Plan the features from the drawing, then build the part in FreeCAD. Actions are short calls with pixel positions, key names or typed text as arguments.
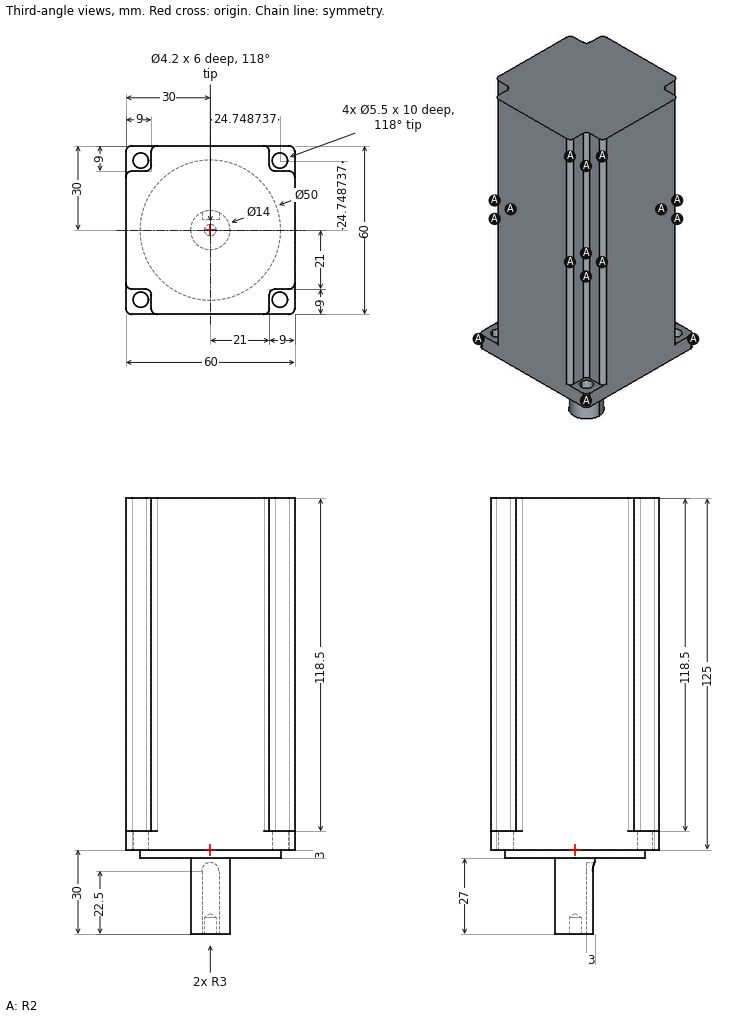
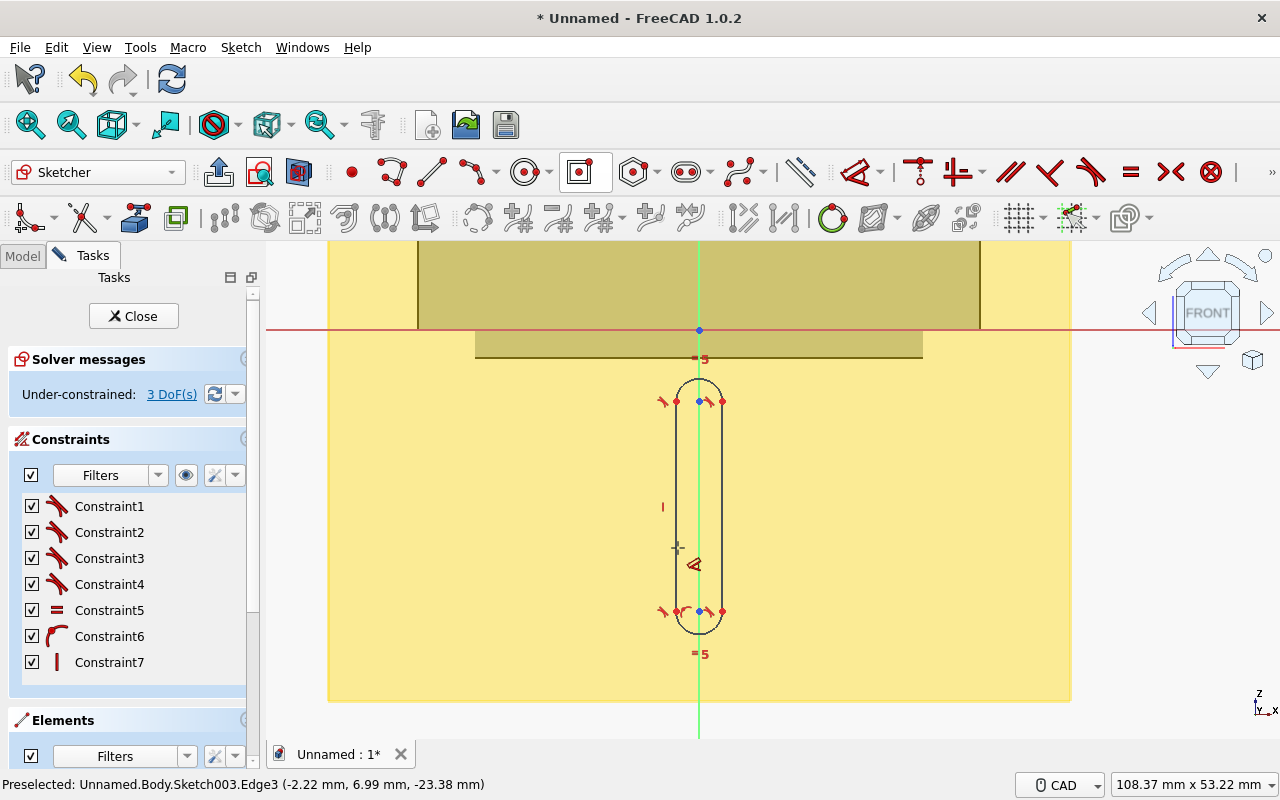
scroll(686, 630, up, 2)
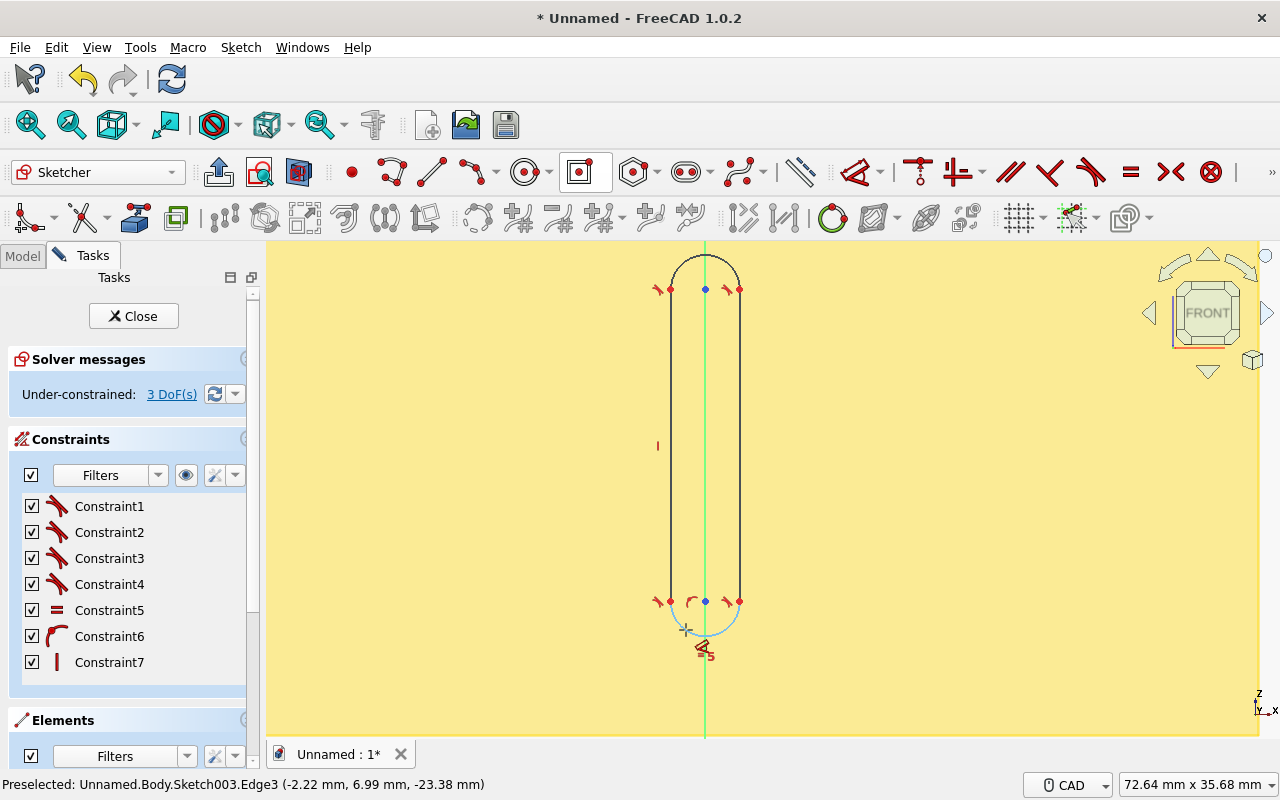
click(685, 630)
click(666, 656)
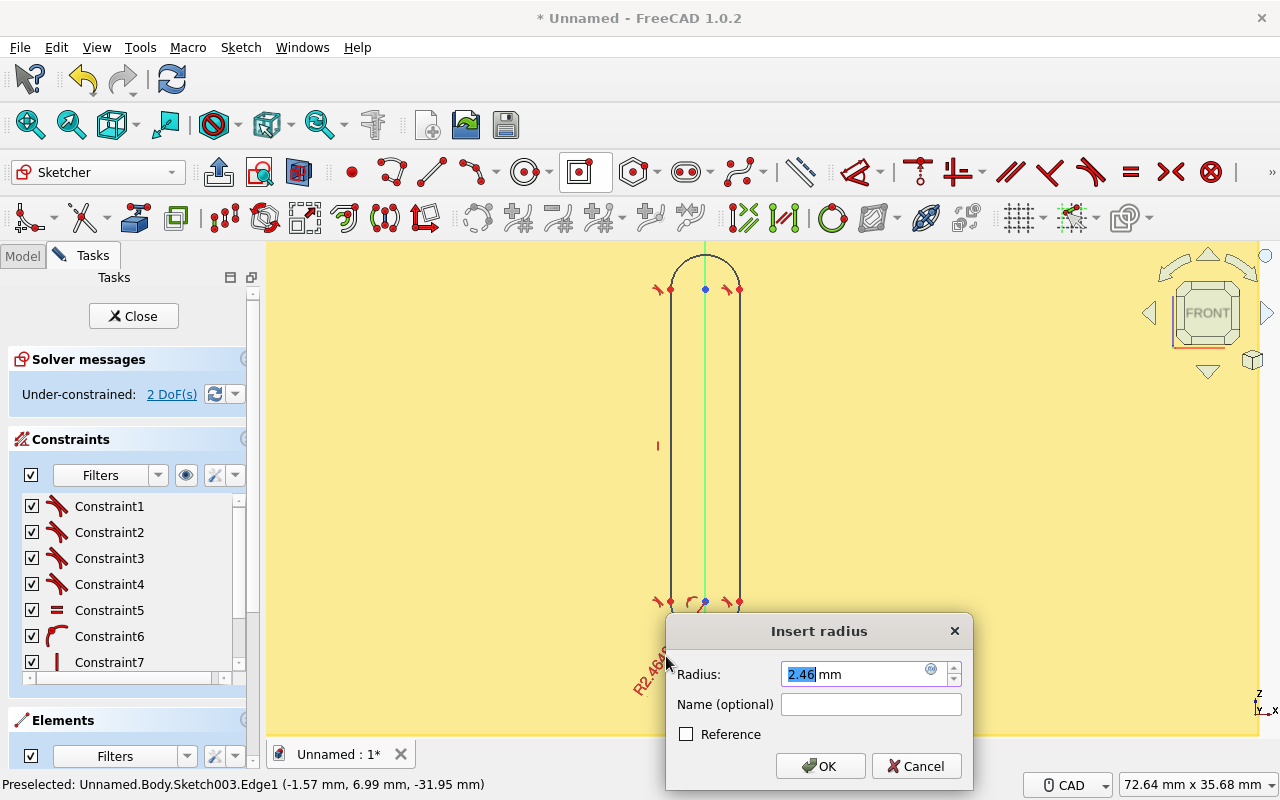
text(3)
key(Return)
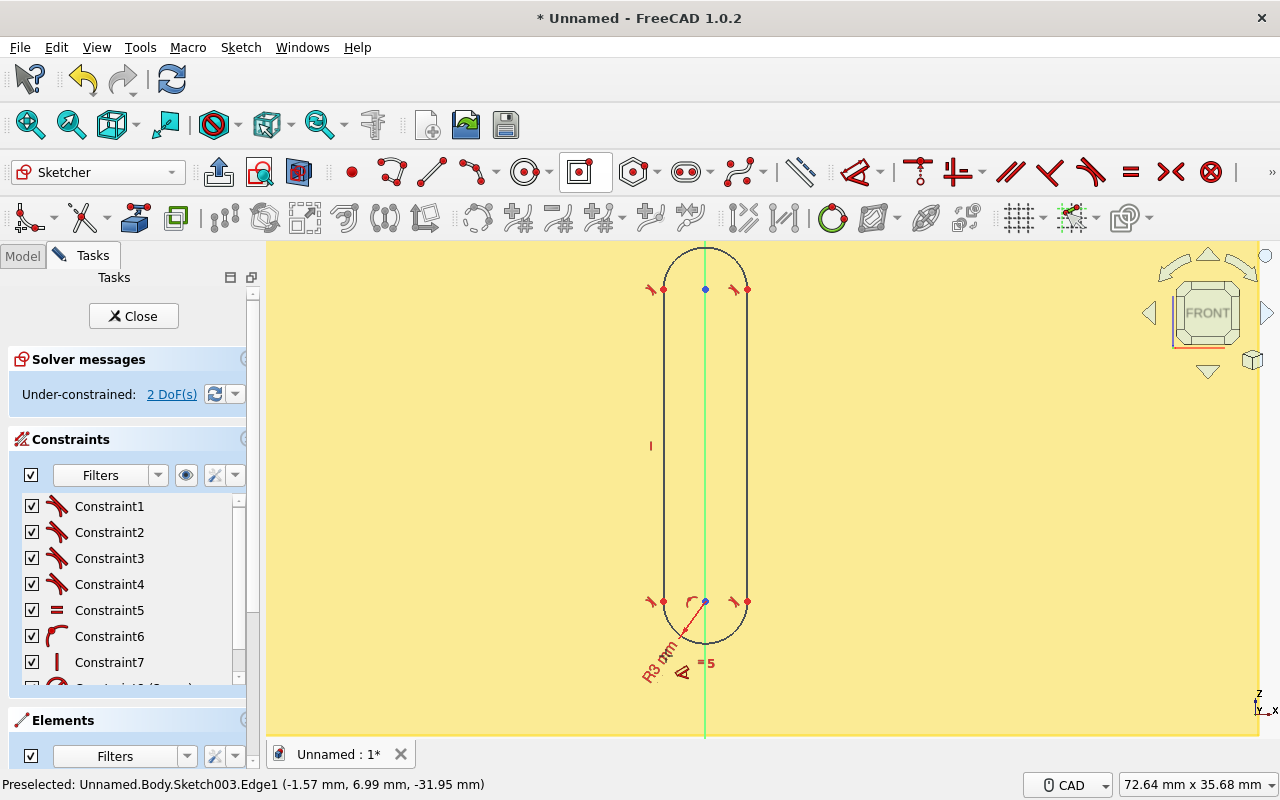
click(664, 602)
click(630, 435)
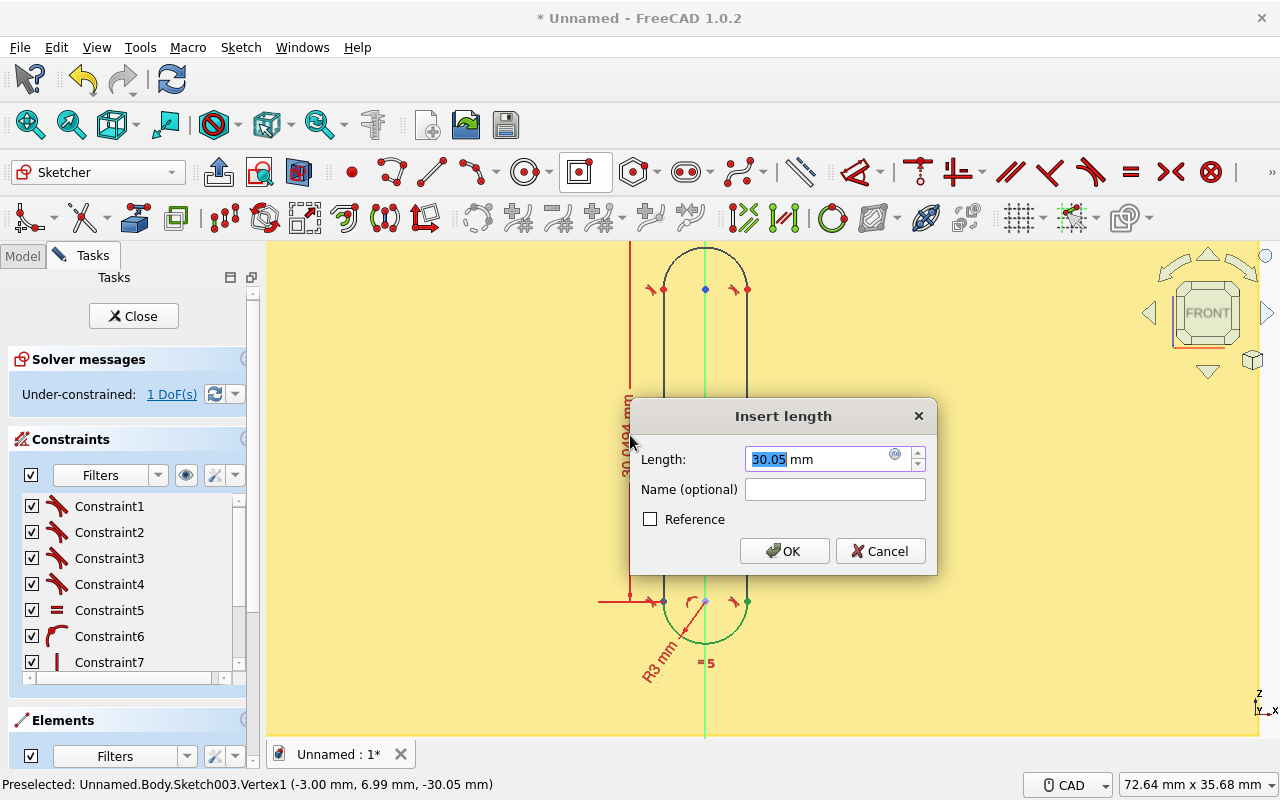
text(30)
key(Return)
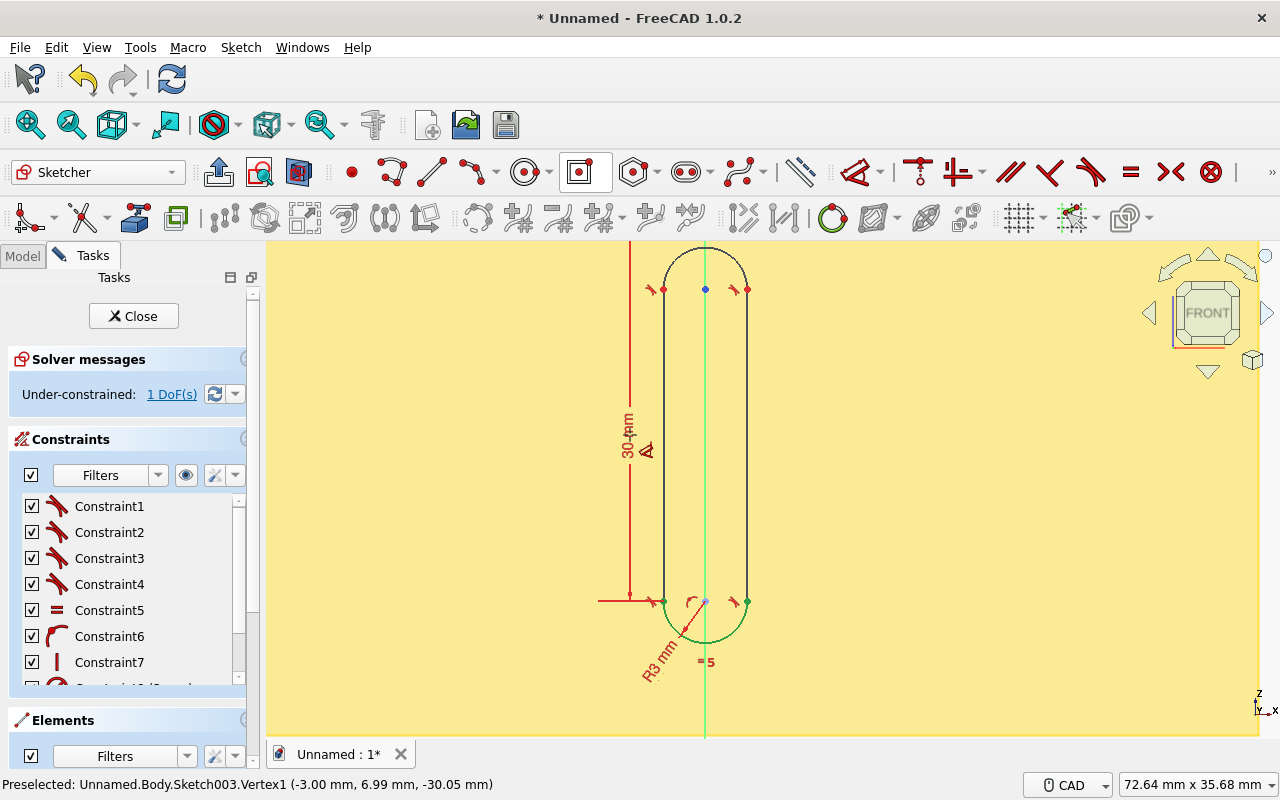
click(664, 508)
click(630, 374)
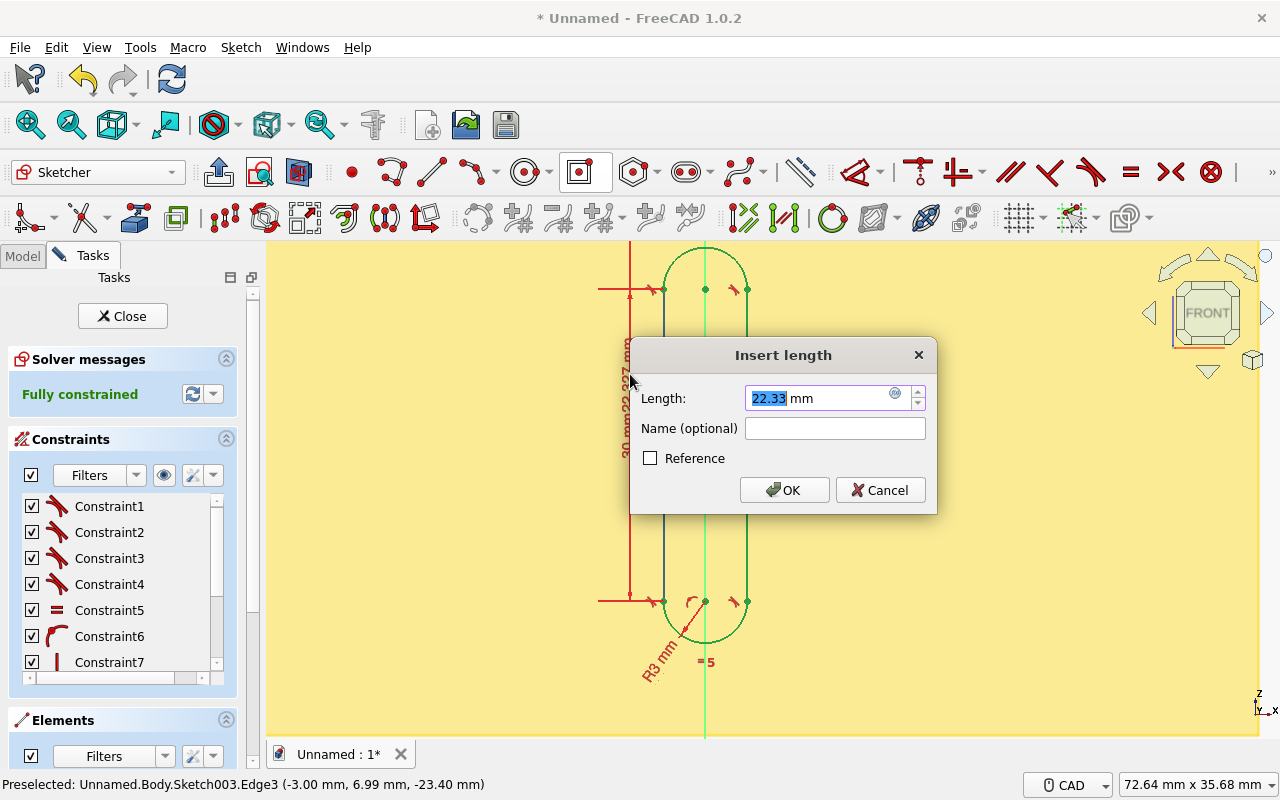
text(22.5)
key(Return)
key(Escape)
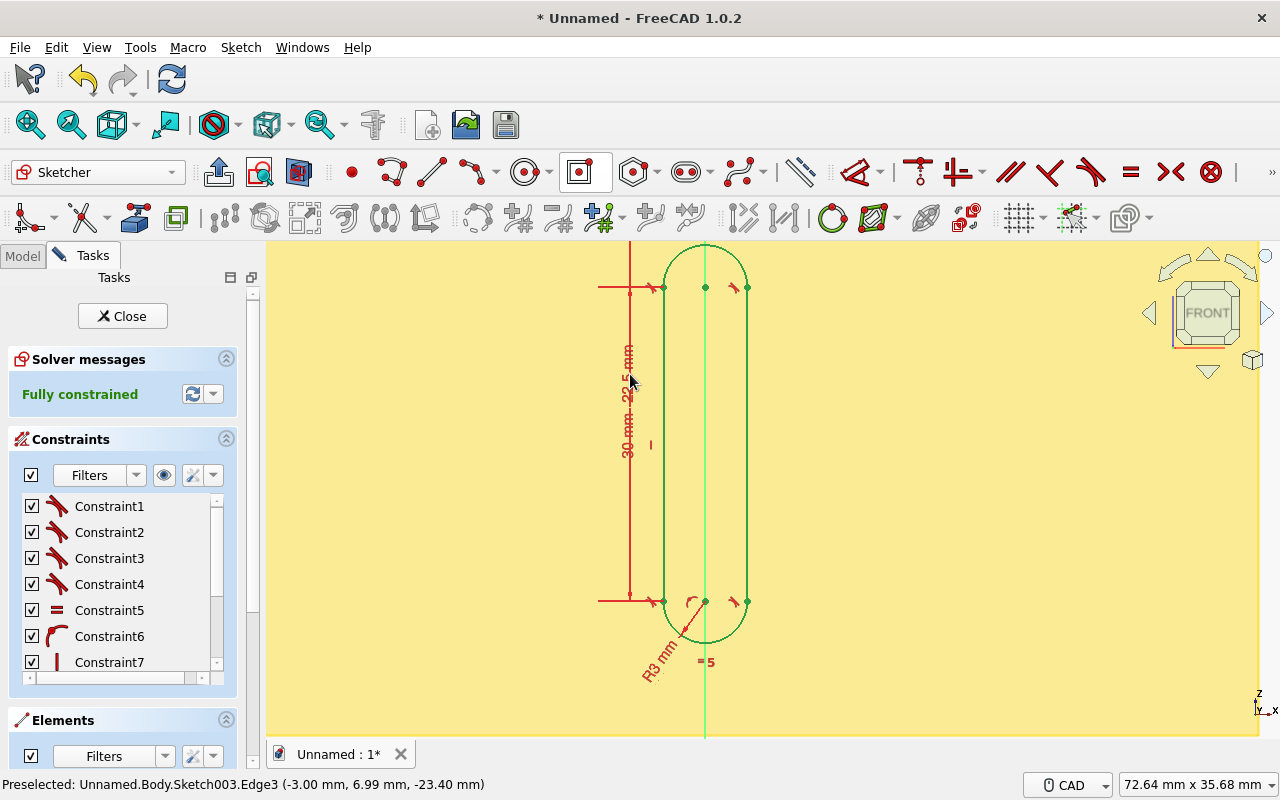
click(123, 316)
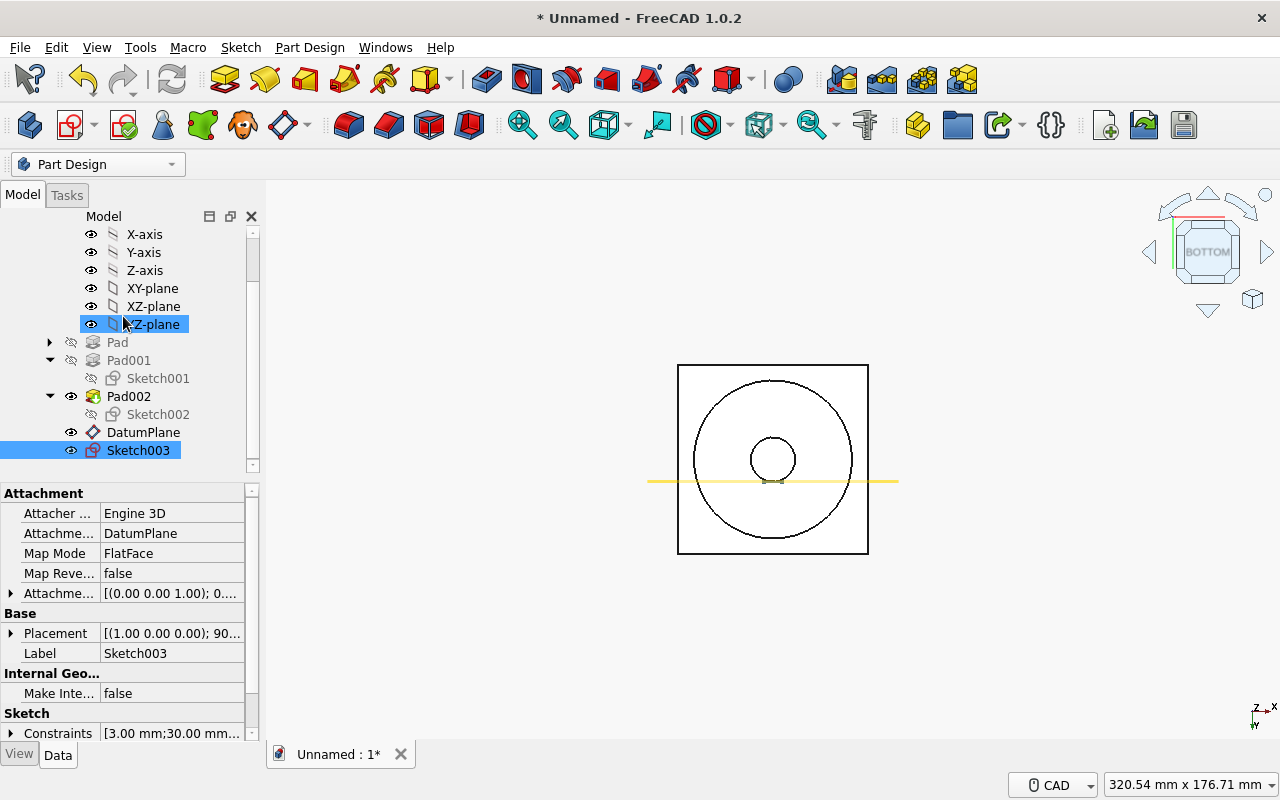
click(488, 80)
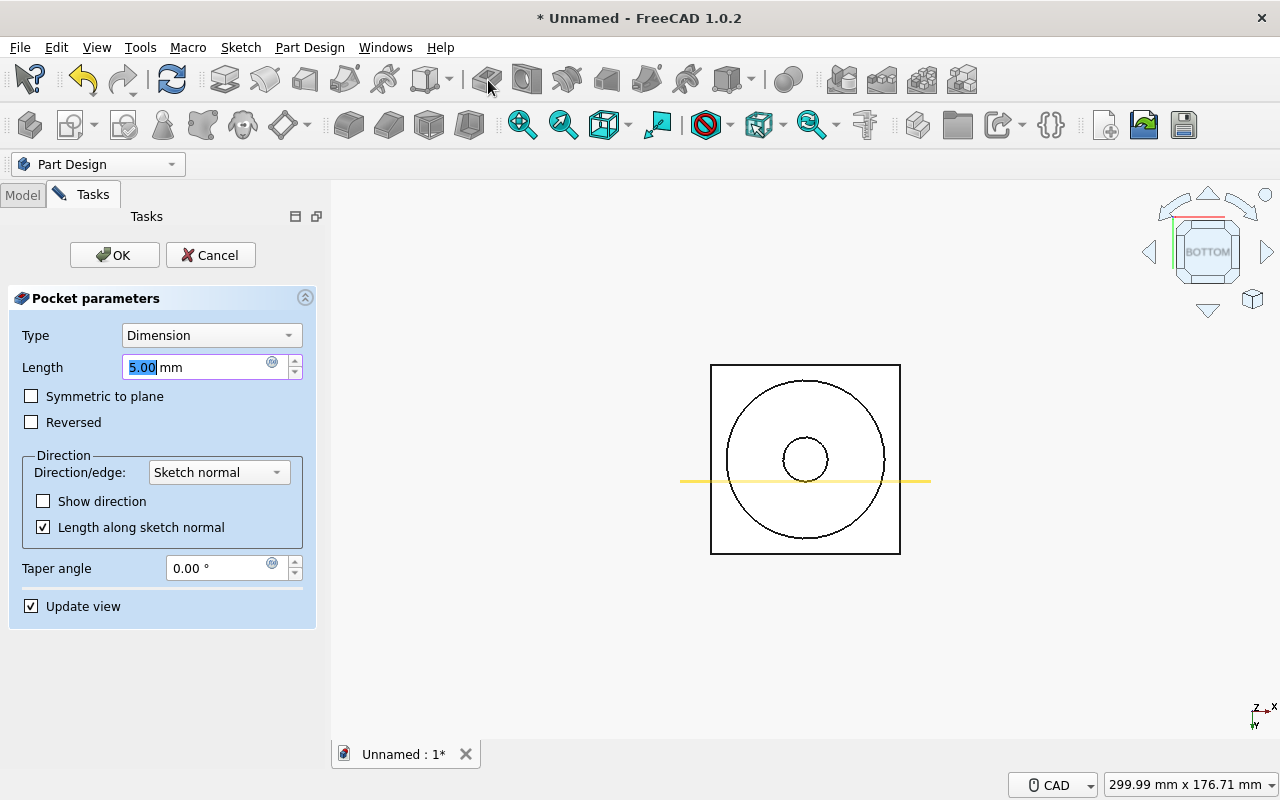
text(3)
key(Tab)